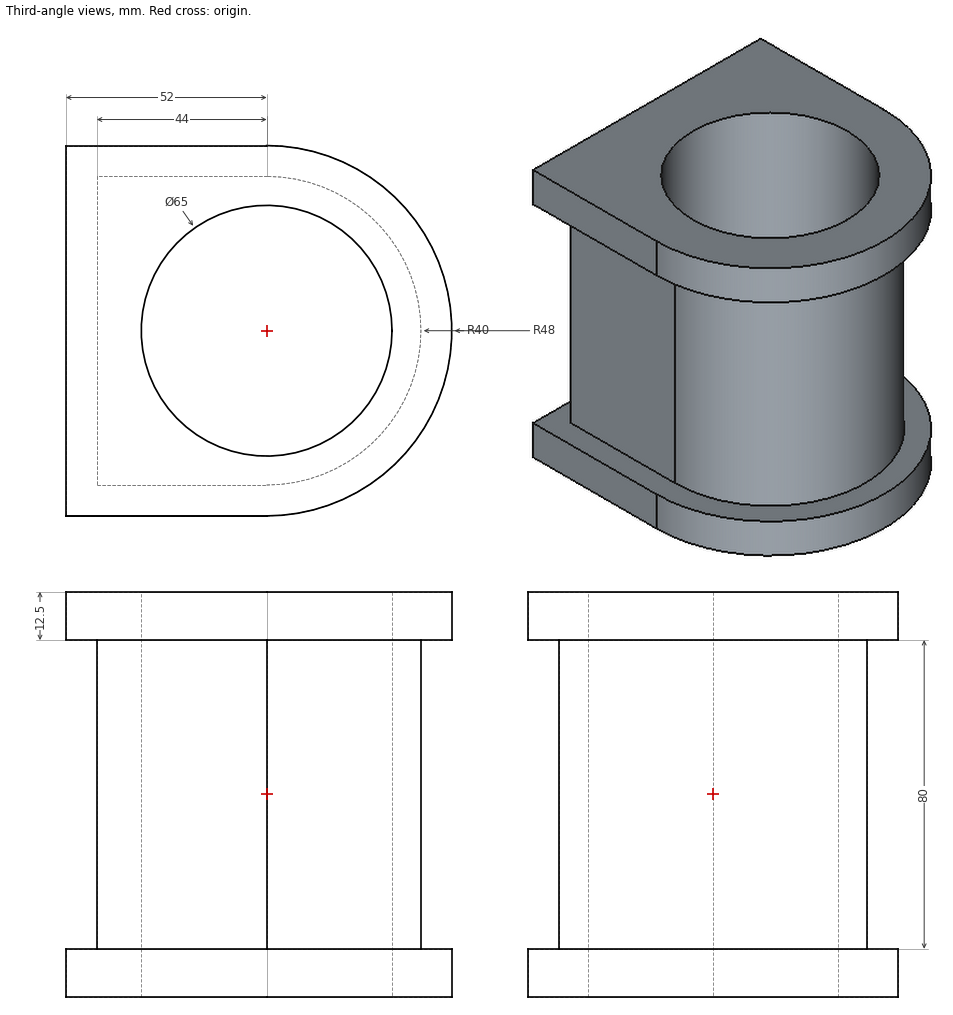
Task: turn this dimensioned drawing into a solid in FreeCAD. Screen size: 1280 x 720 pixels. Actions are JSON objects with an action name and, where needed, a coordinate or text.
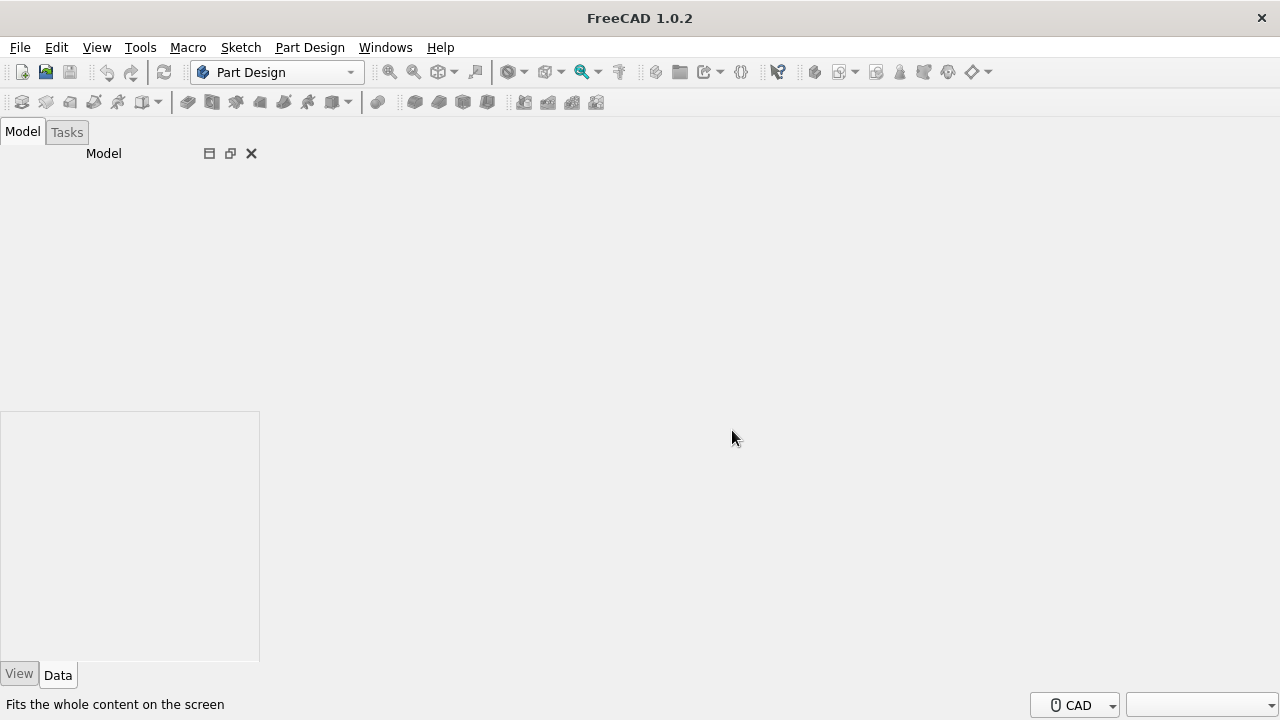
{"action": "left_click", "coordinate": [22, 72]}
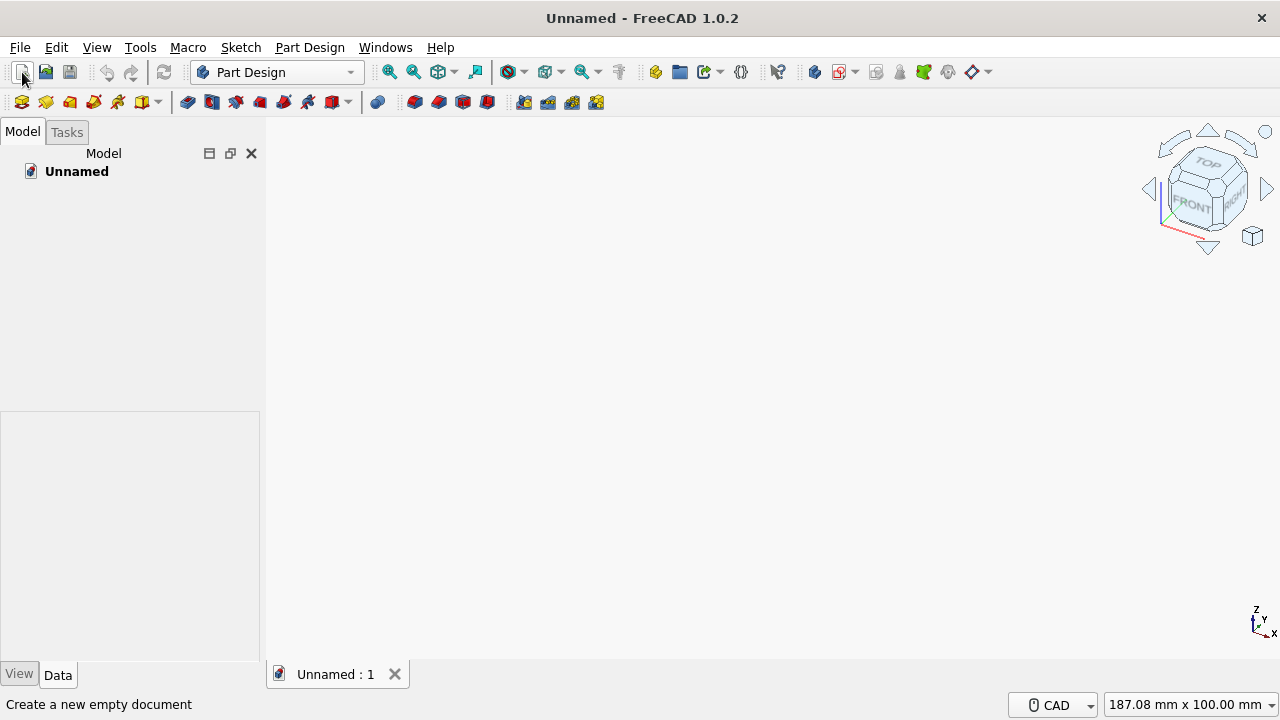
{"action": "left_click", "coordinate": [840, 72]}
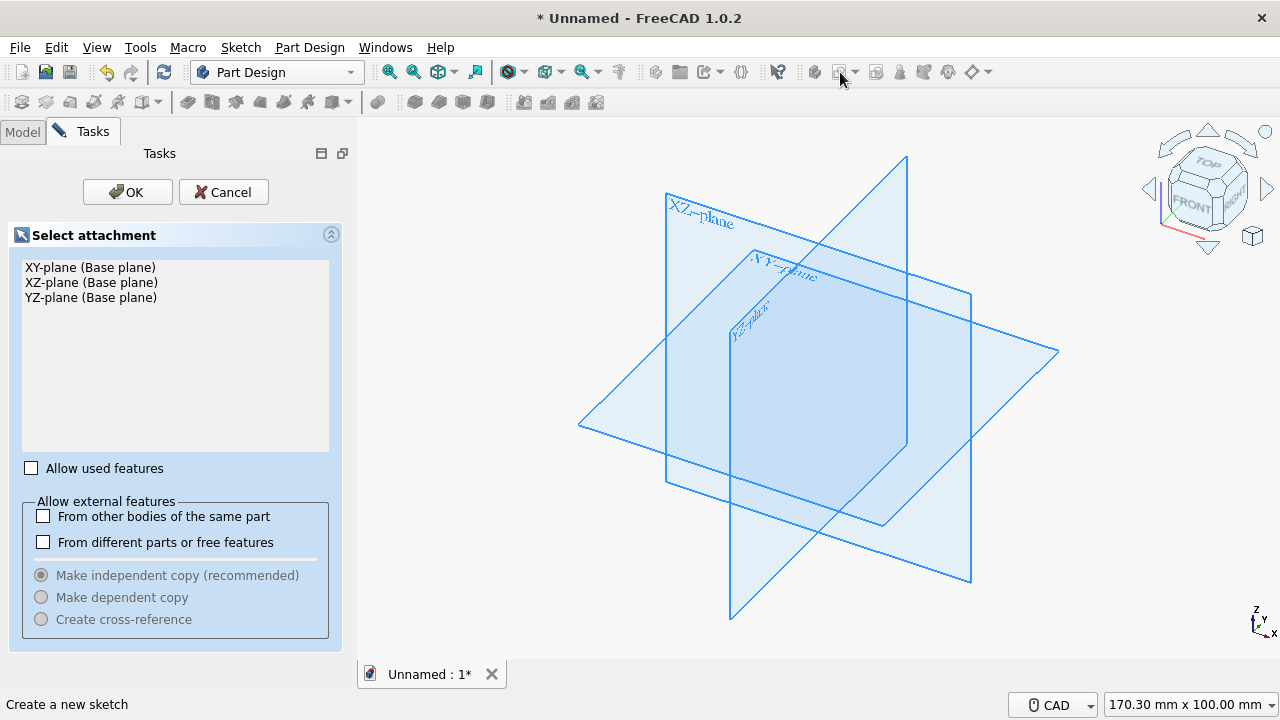
{"action": "left_click", "coordinate": [82, 268]}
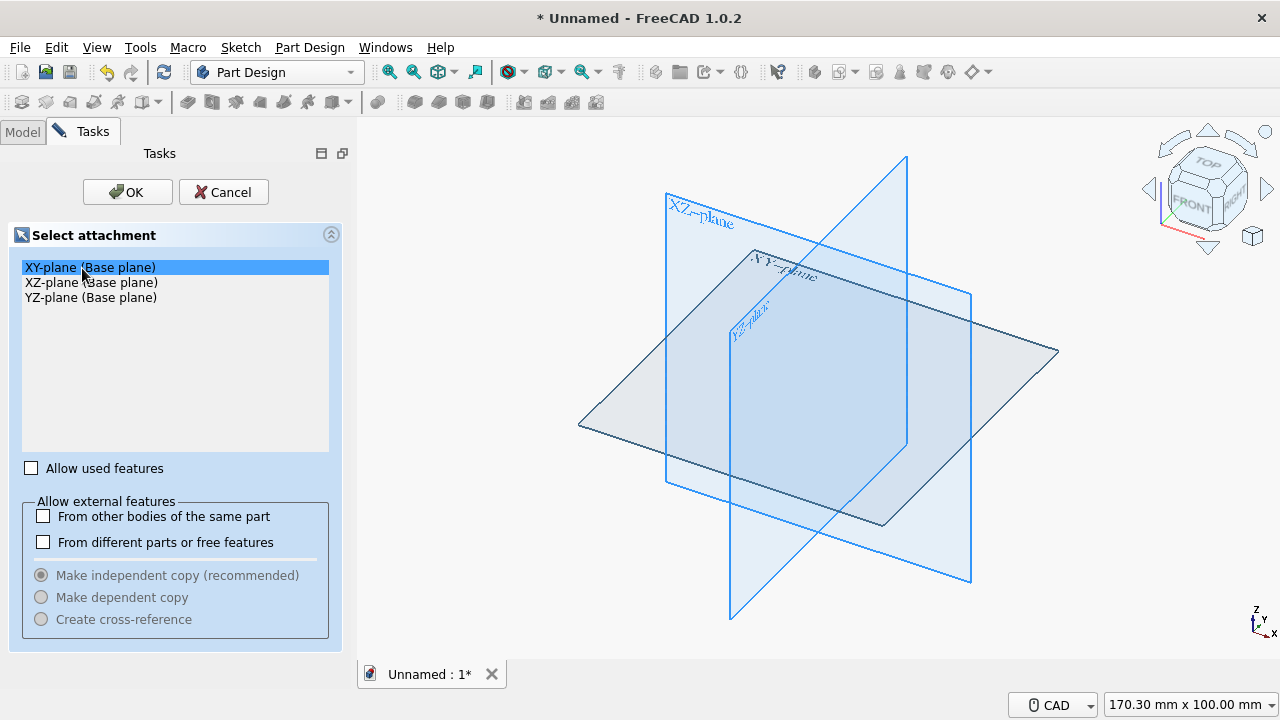
{"action": "left_click", "coordinate": [128, 192]}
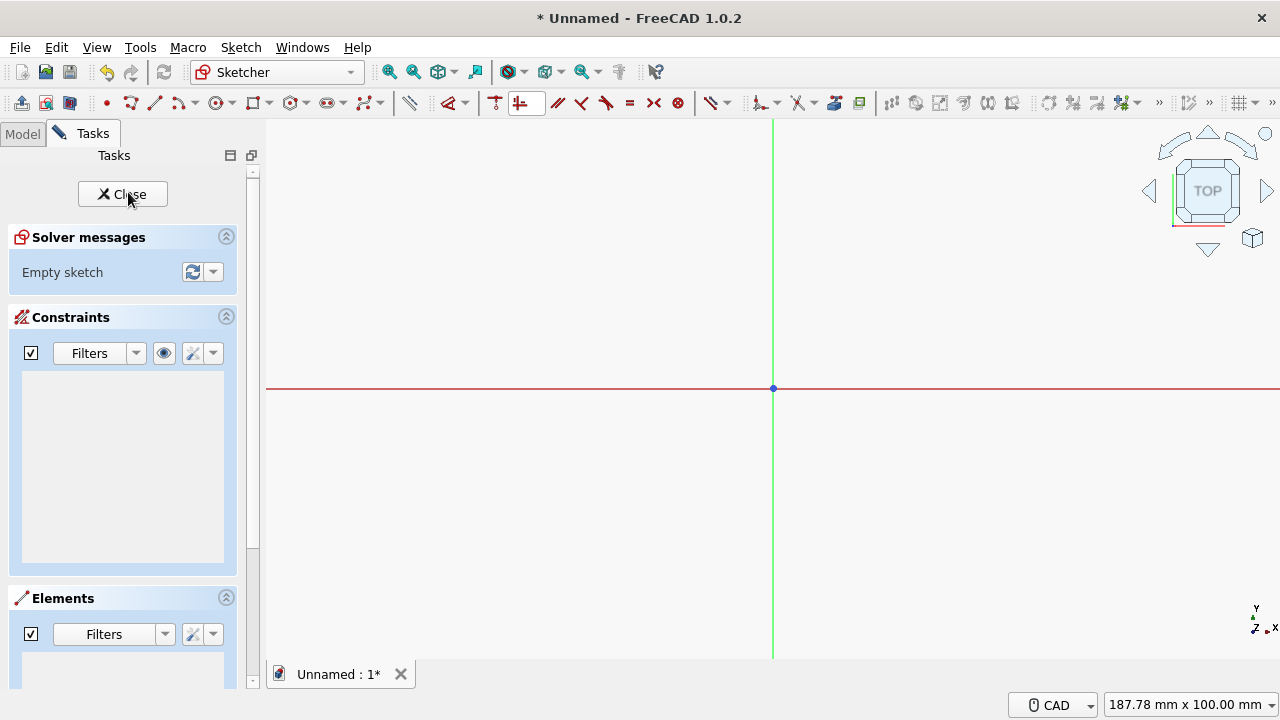
{"action": "left_click", "coordinate": [132, 104]}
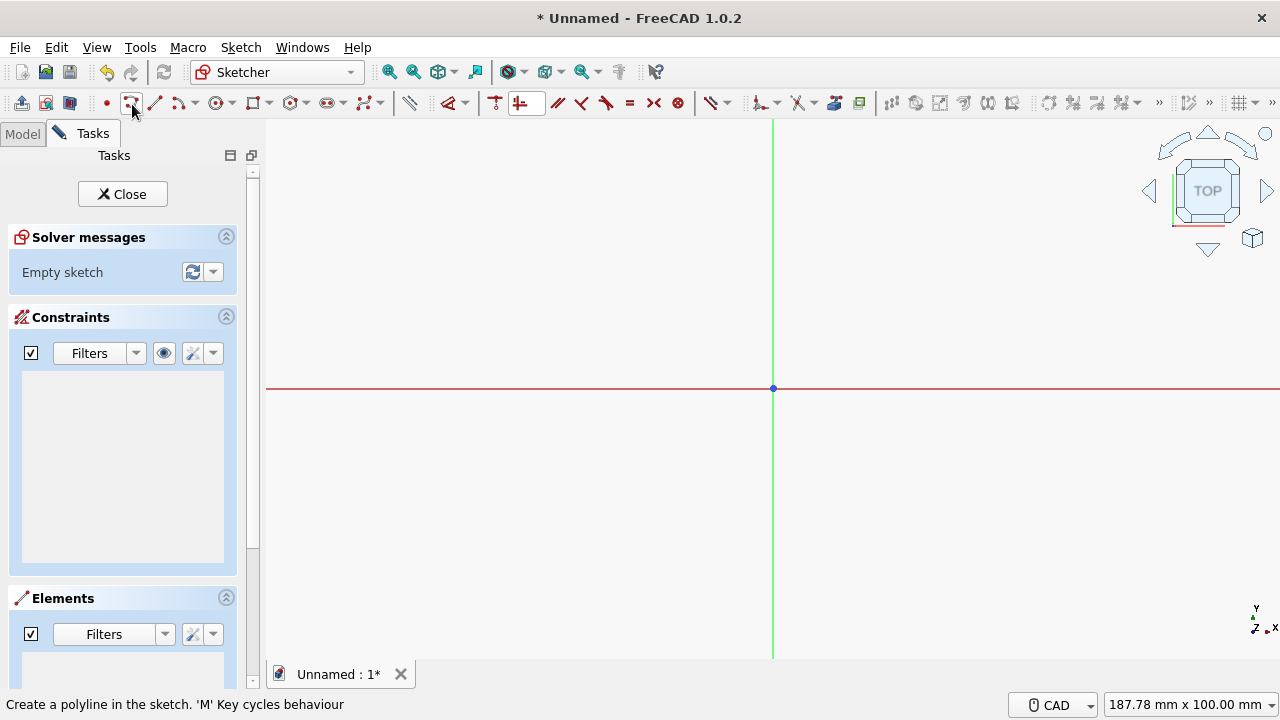
{"action": "left_click", "coordinate": [773, 173]}
{"action": "left_click", "coordinate": [535, 173]}
{"action": "left_click", "coordinate": [535, 605]}
{"action": "left_click", "coordinate": [773, 605]}
{"action": "right_click", "coordinate": [773, 605]}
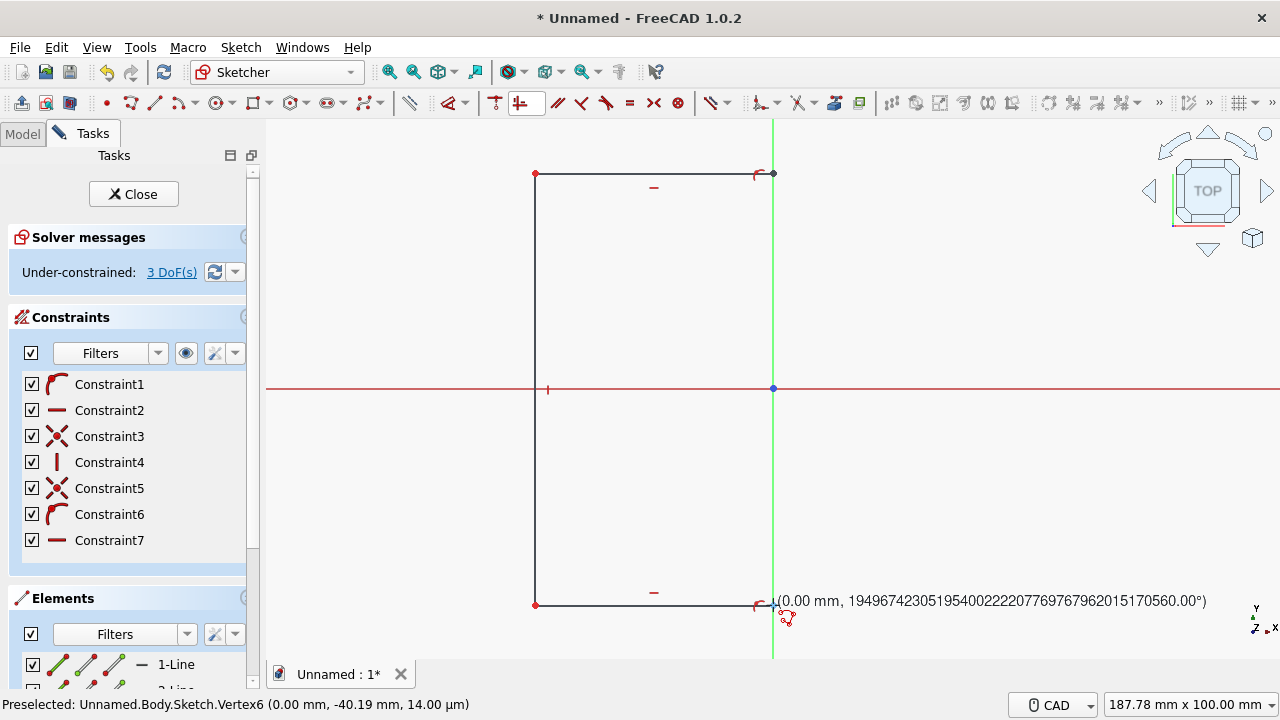
{"action": "key", "text": "g 3 a"}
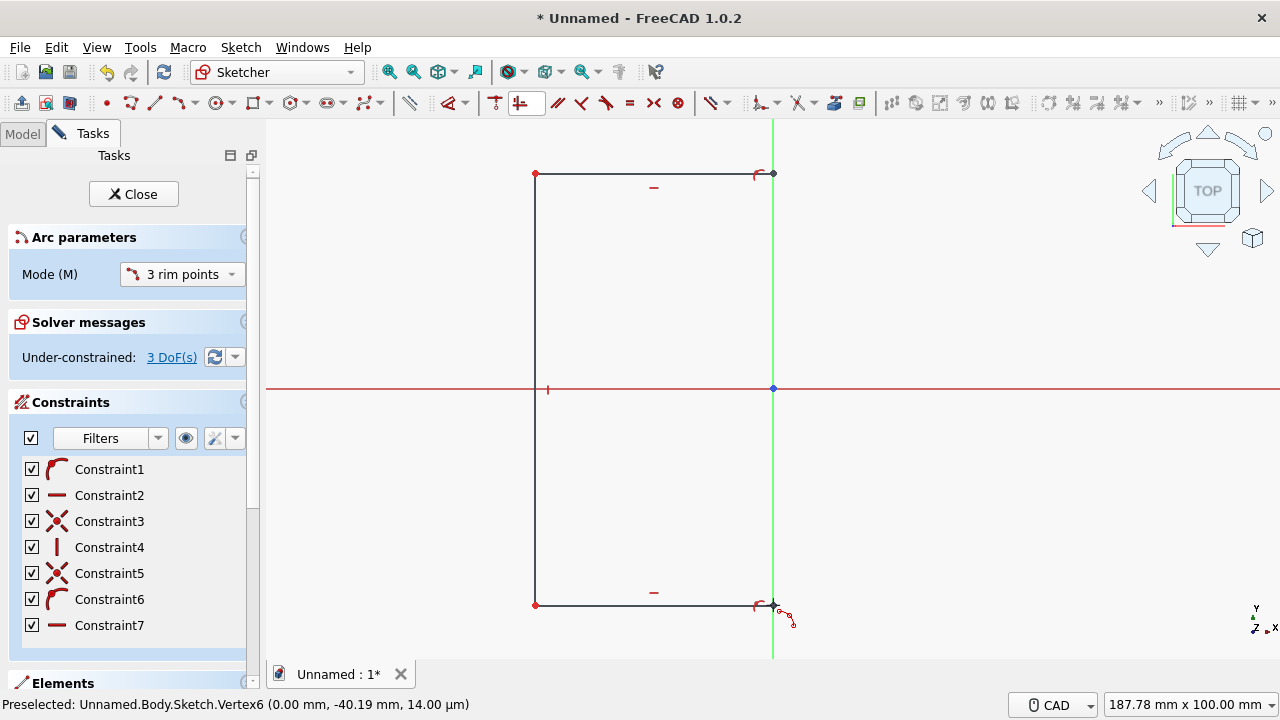
{"action": "left_click", "coordinate": [773, 606]}
{"action": "left_click", "coordinate": [773, 174]}
{"action": "left_click", "coordinate": [978, 456]}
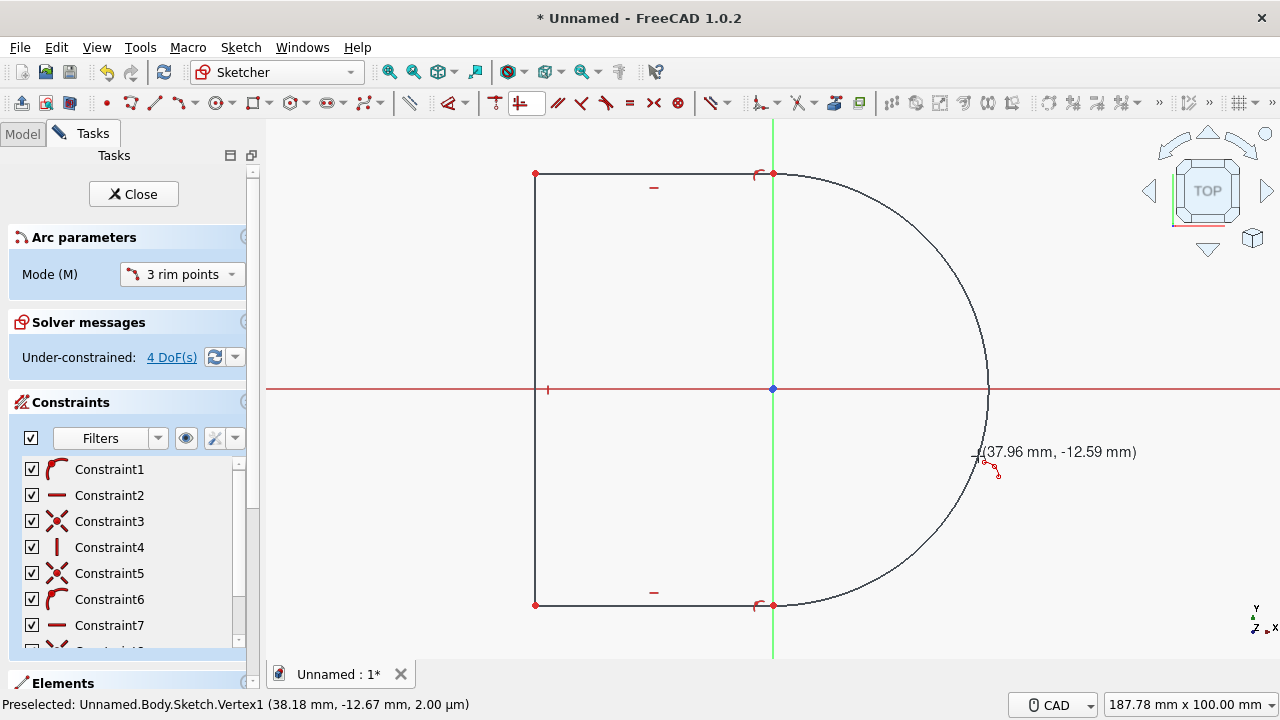
{"action": "left_click", "coordinate": [216, 104]}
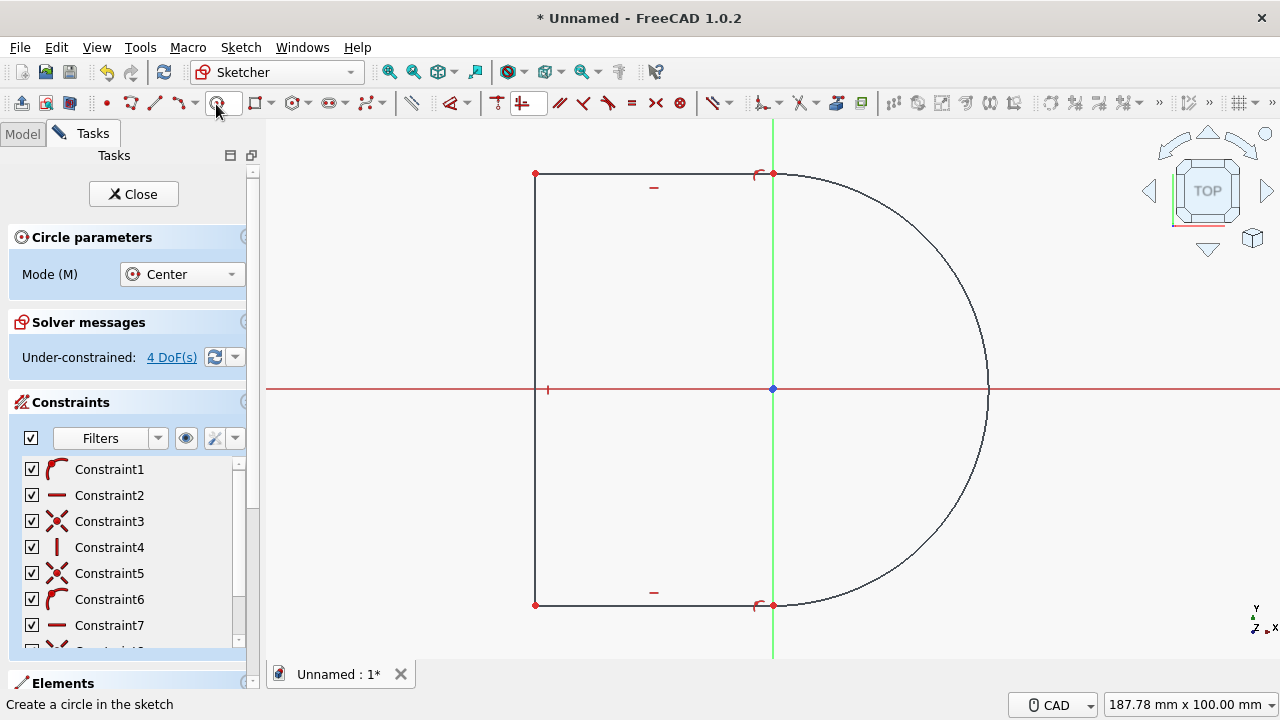
{"action": "left_click", "coordinate": [773, 389]}
{"action": "left_click", "coordinate": [897, 265]}
{"action": "key", "text": "Escape"}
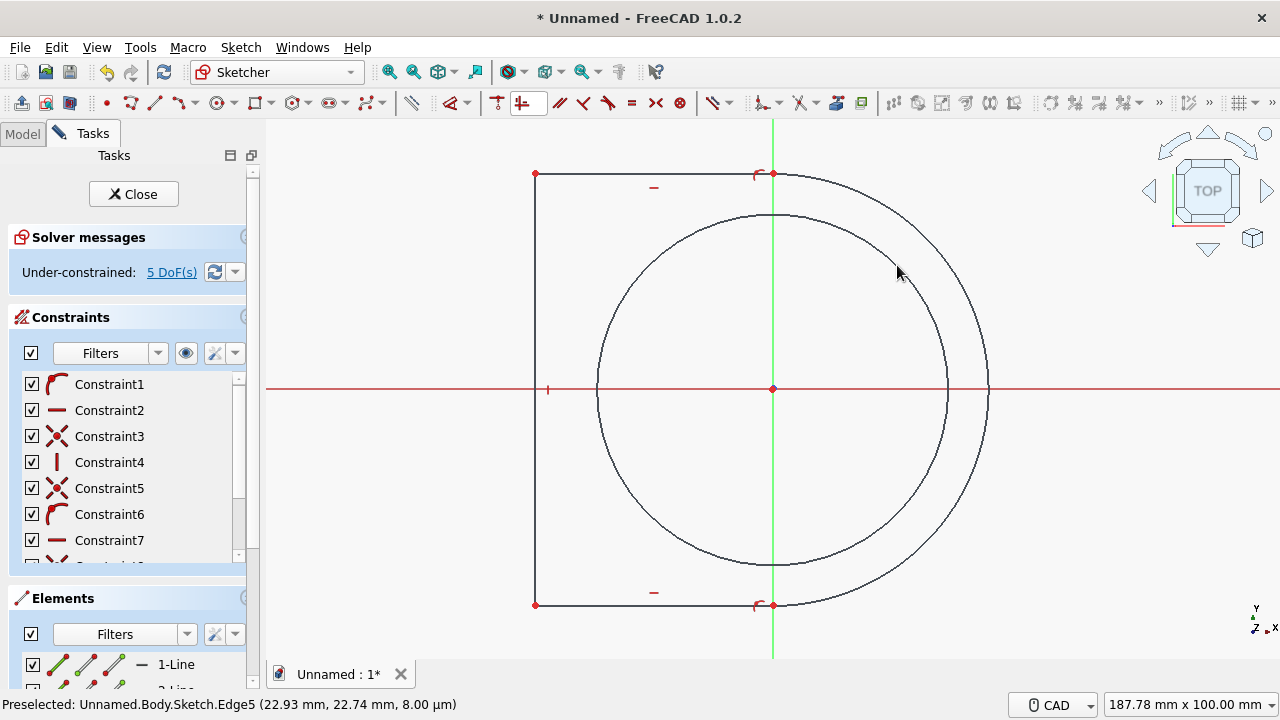
{"action": "left_click_drag", "start_coordinate": [763, 379], "coordinate": [783, 400]}